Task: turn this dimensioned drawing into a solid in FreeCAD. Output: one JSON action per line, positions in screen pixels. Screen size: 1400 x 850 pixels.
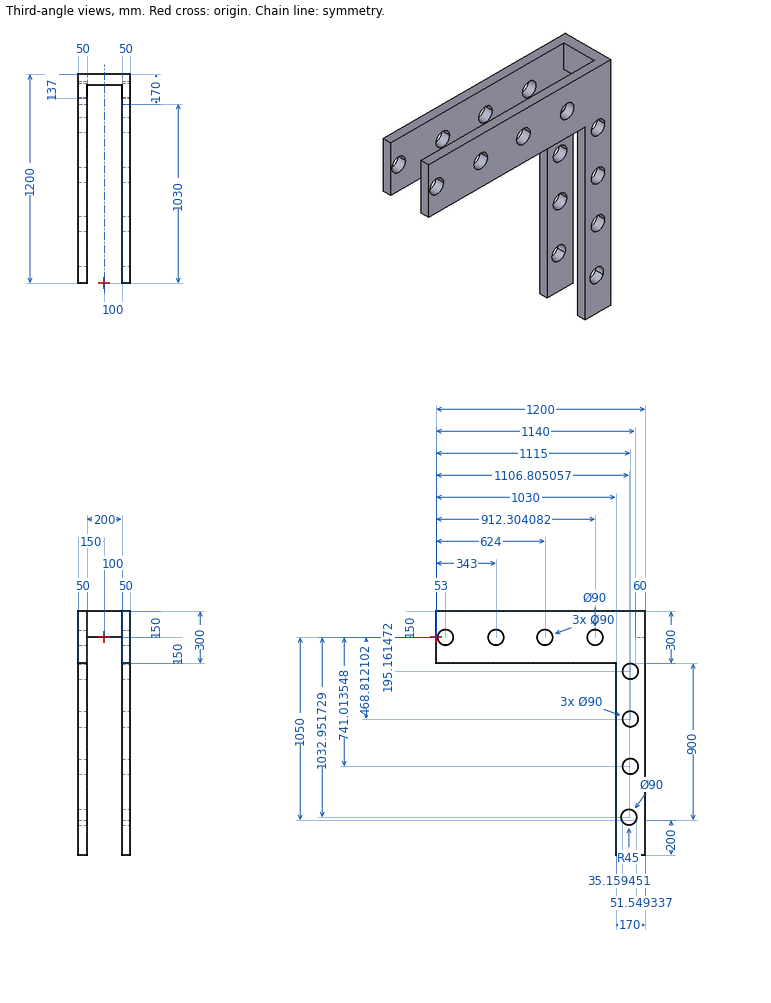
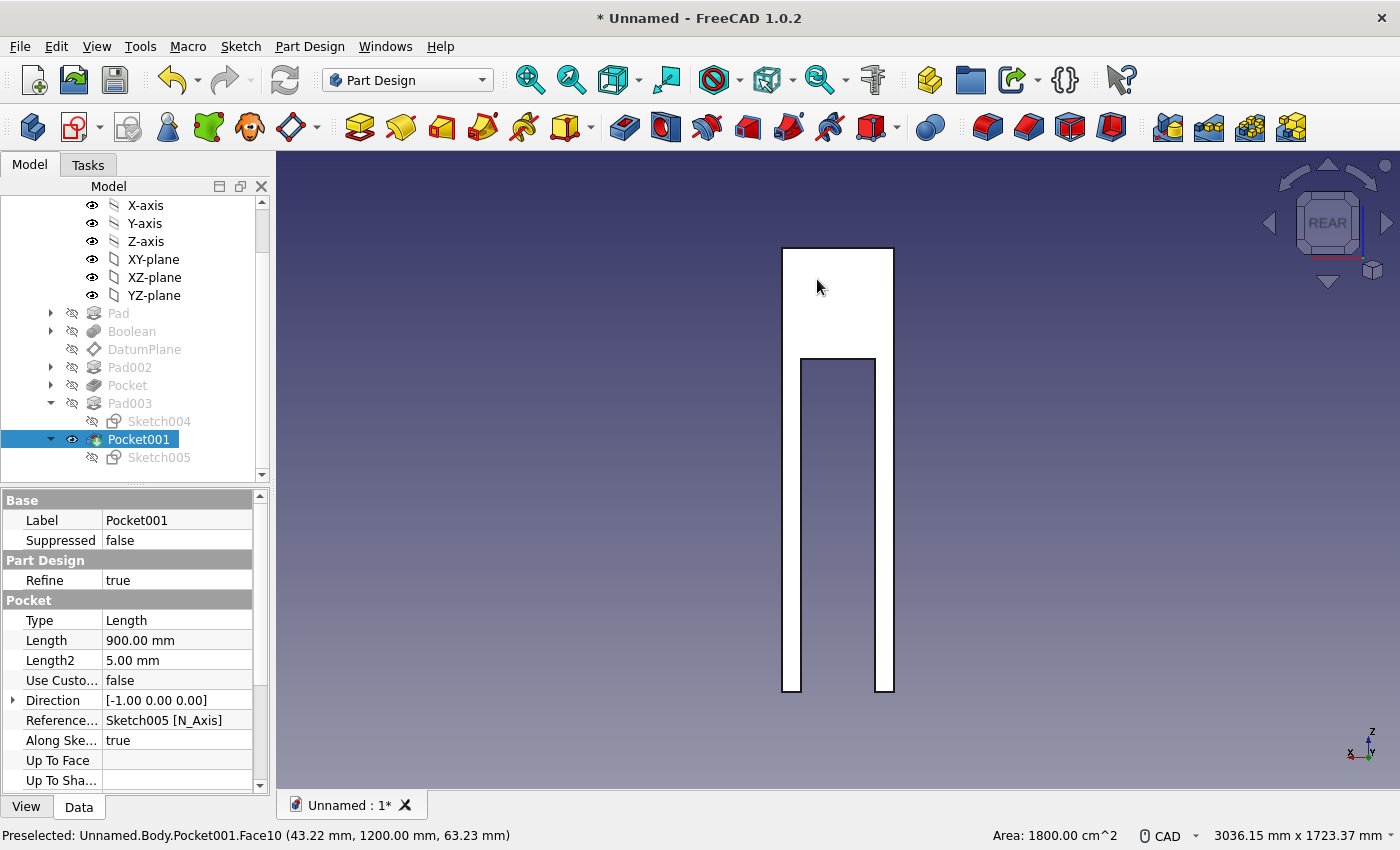
{"action": "left_click", "coordinate": [74, 128]}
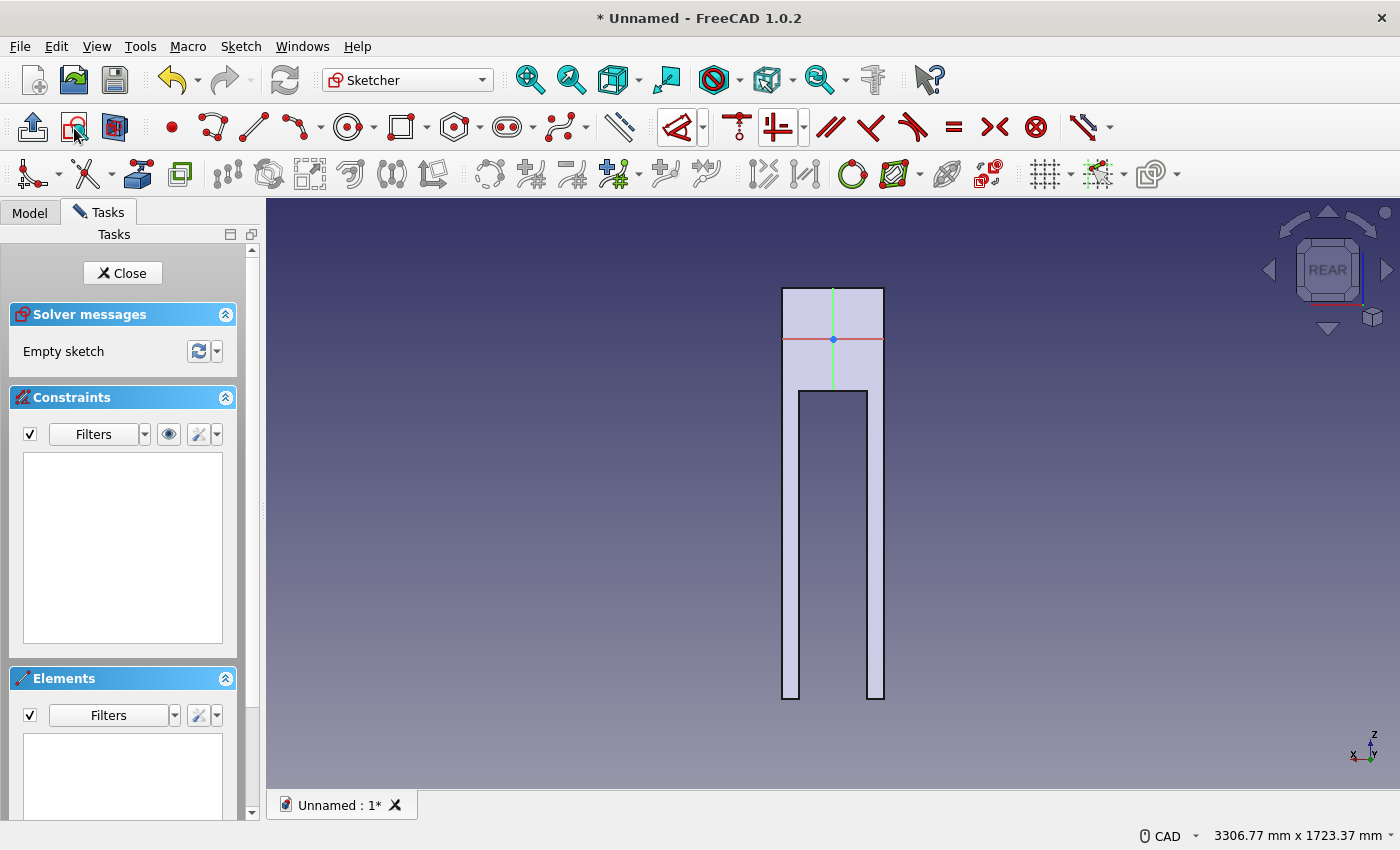
{"action": "scroll", "coordinate": [844, 345], "scroll_direction": "up", "scroll_amount": 10}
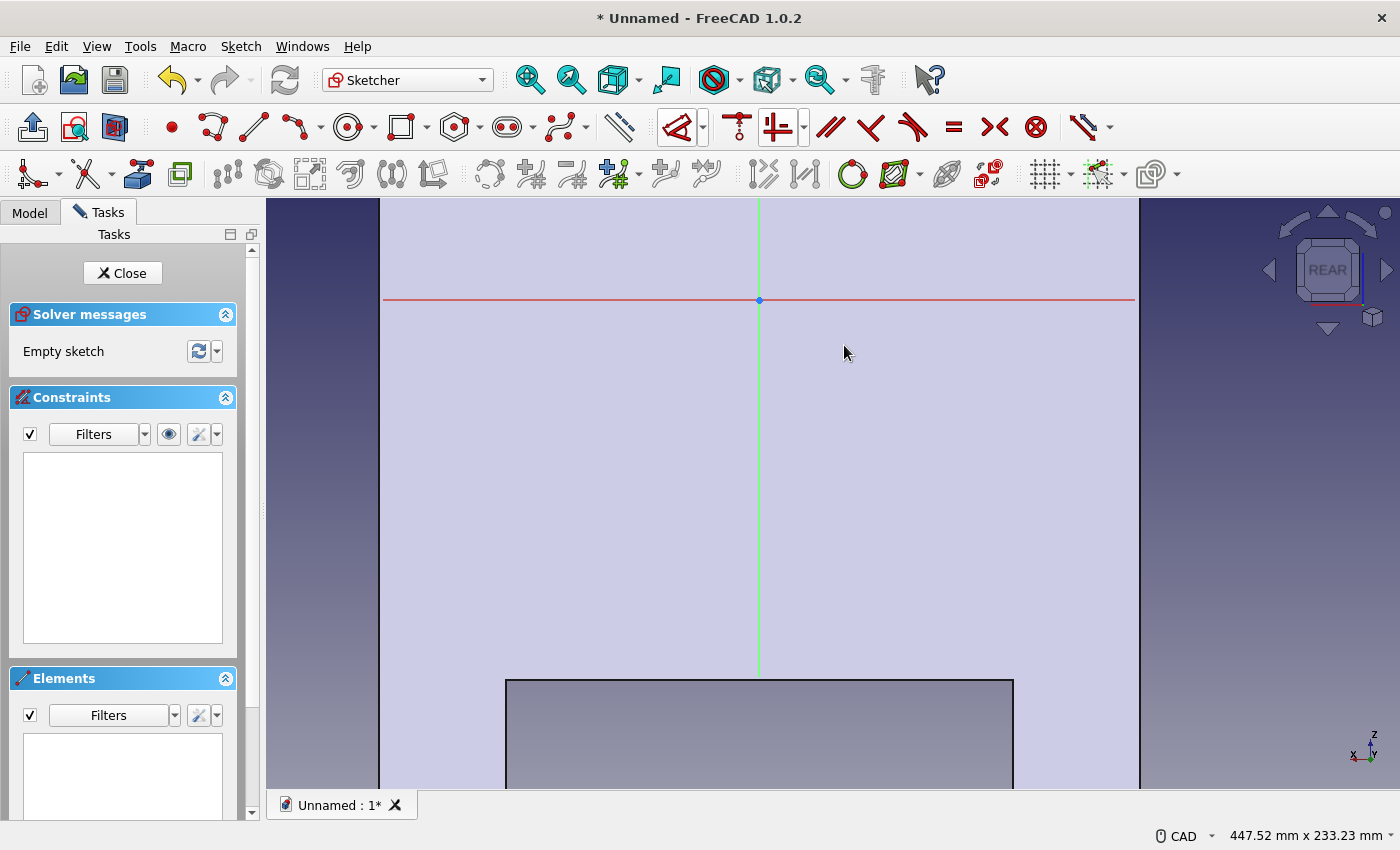
{"action": "left_click", "coordinate": [400, 128]}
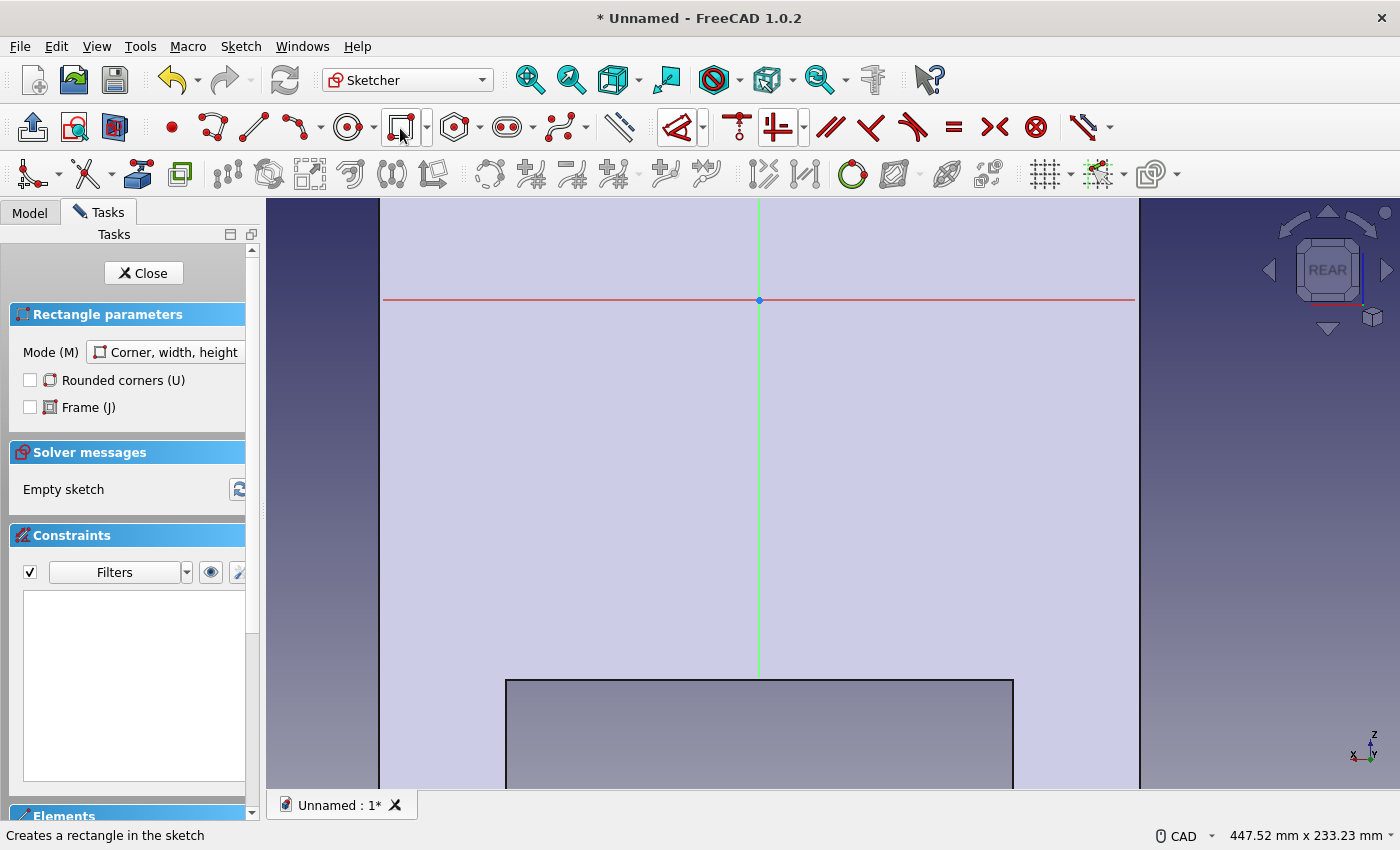
{"action": "left_click", "coordinate": [506, 300]}
{"action": "left_click", "coordinate": [1013, 680]}
{"action": "key", "text": "Escape"}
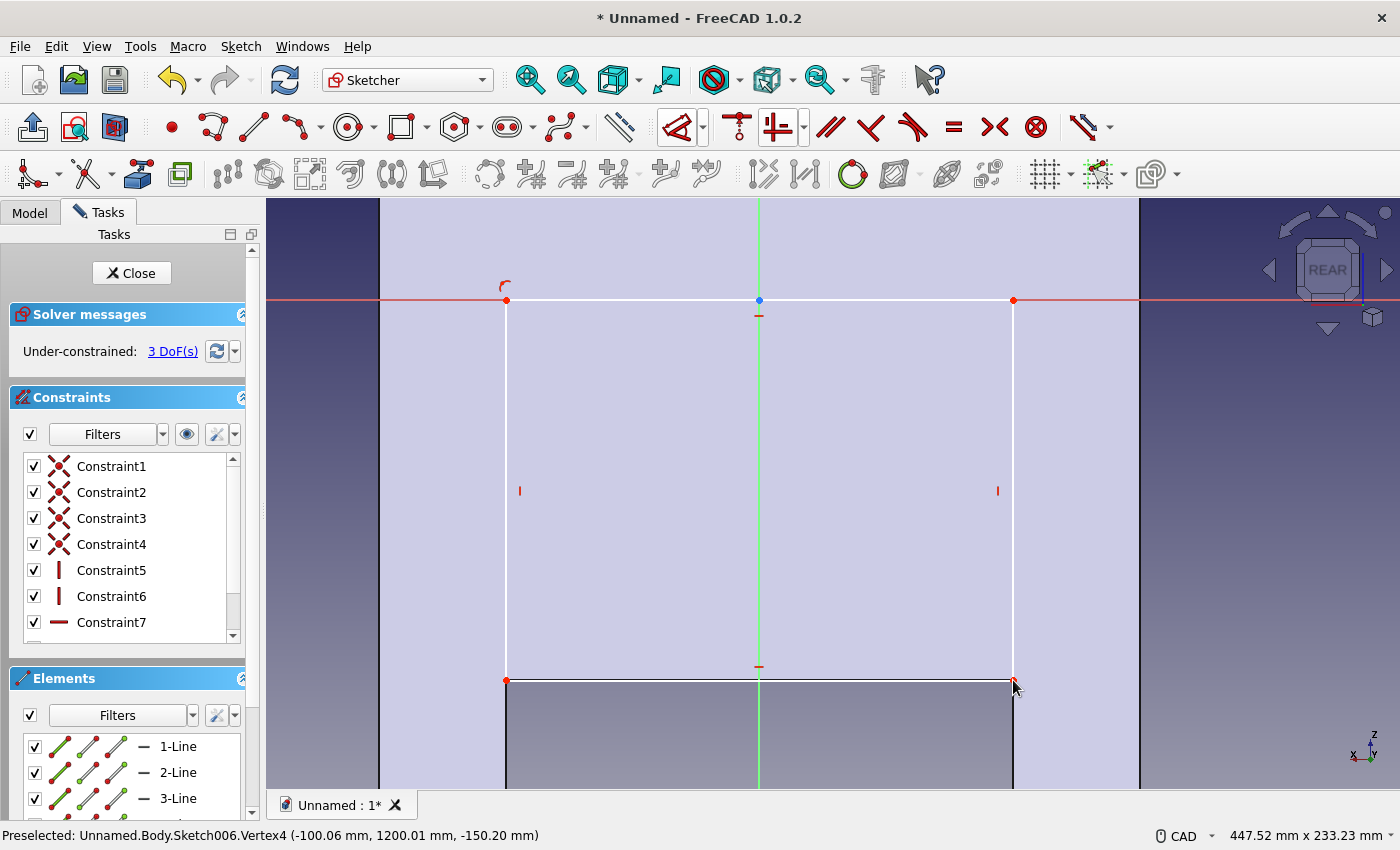
{"action": "left_click", "coordinate": [506, 415]}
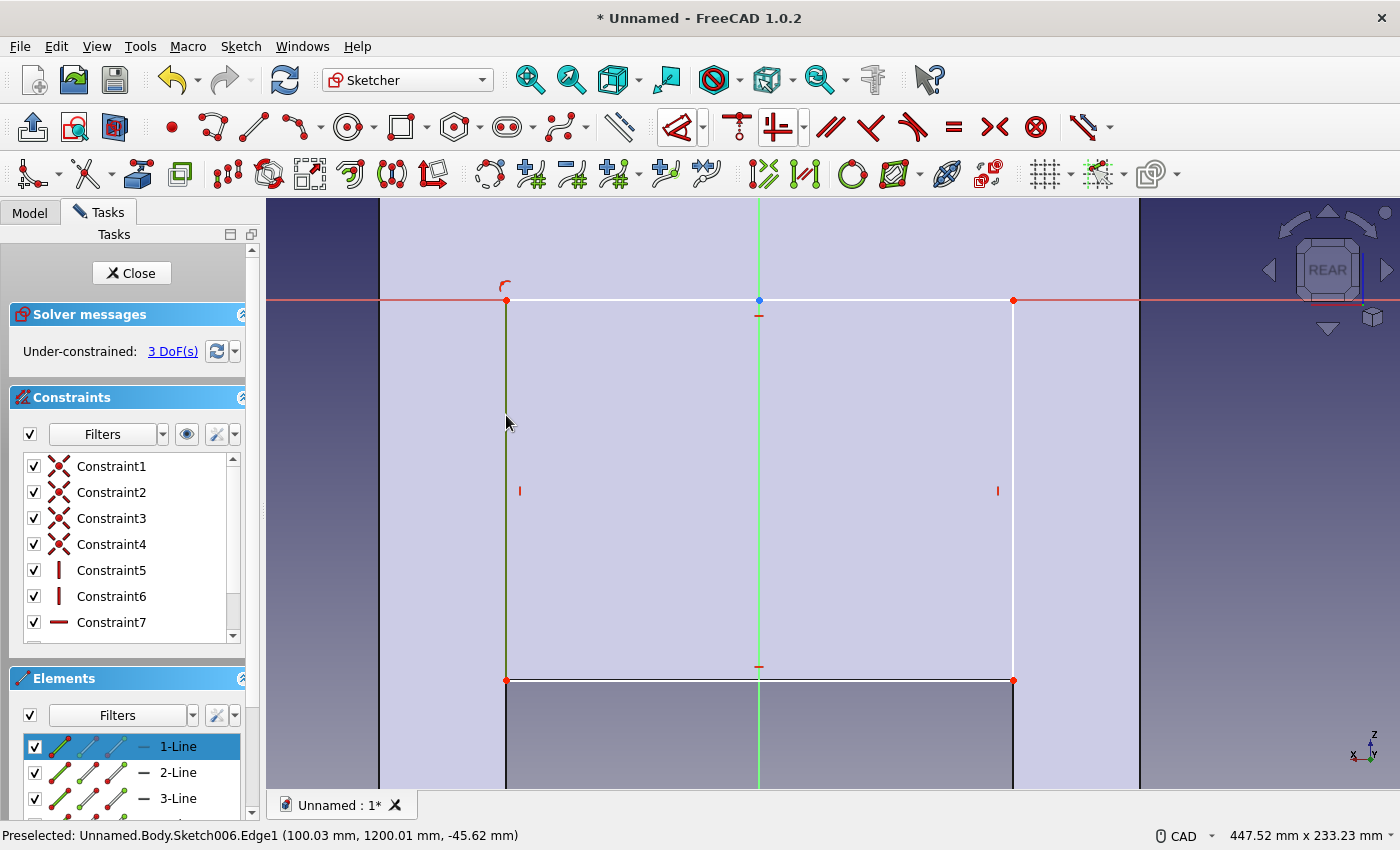
{"action": "key", "text": "i"}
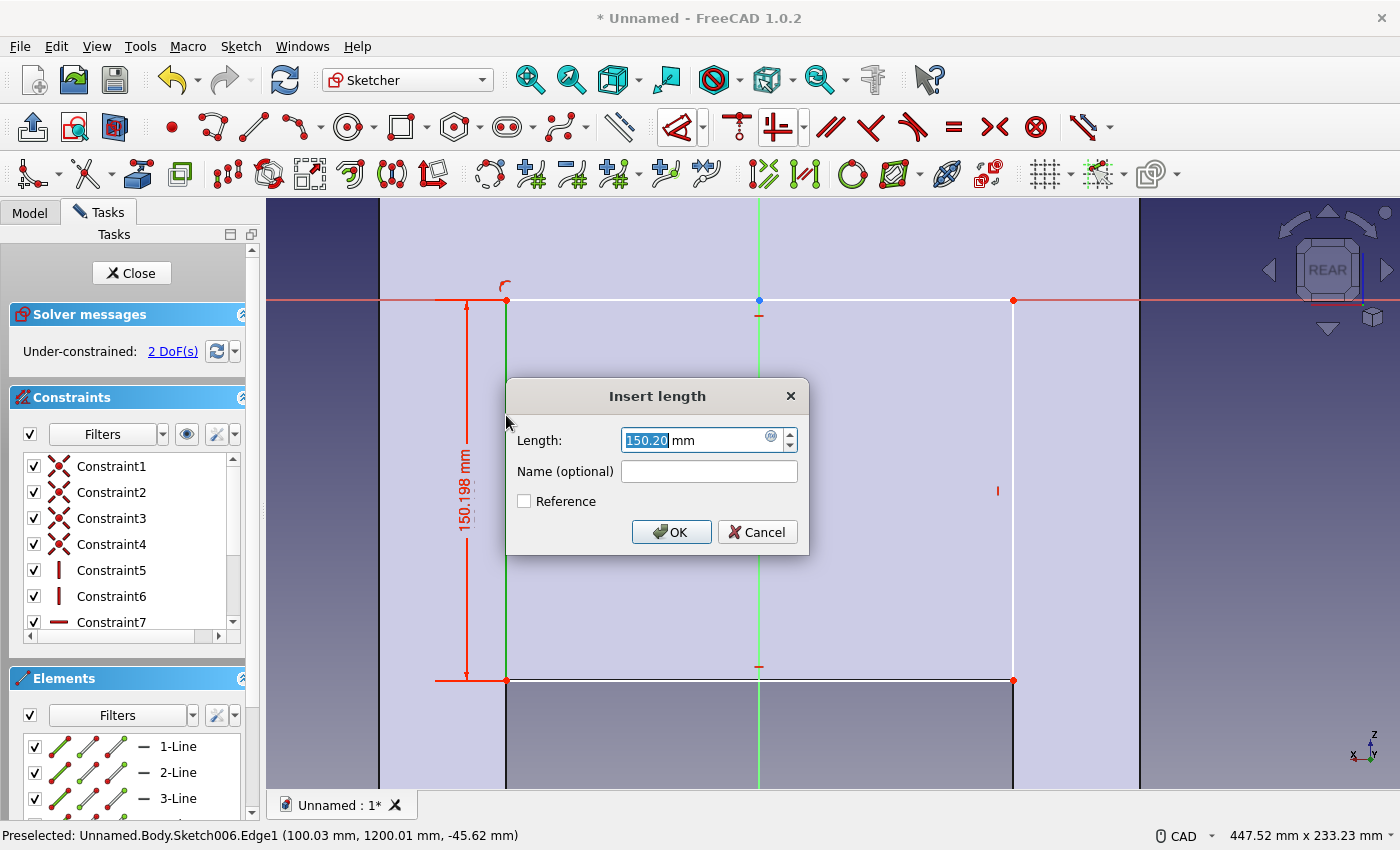
{"action": "type", "text": "150"}
{"action": "key", "text": "Return"}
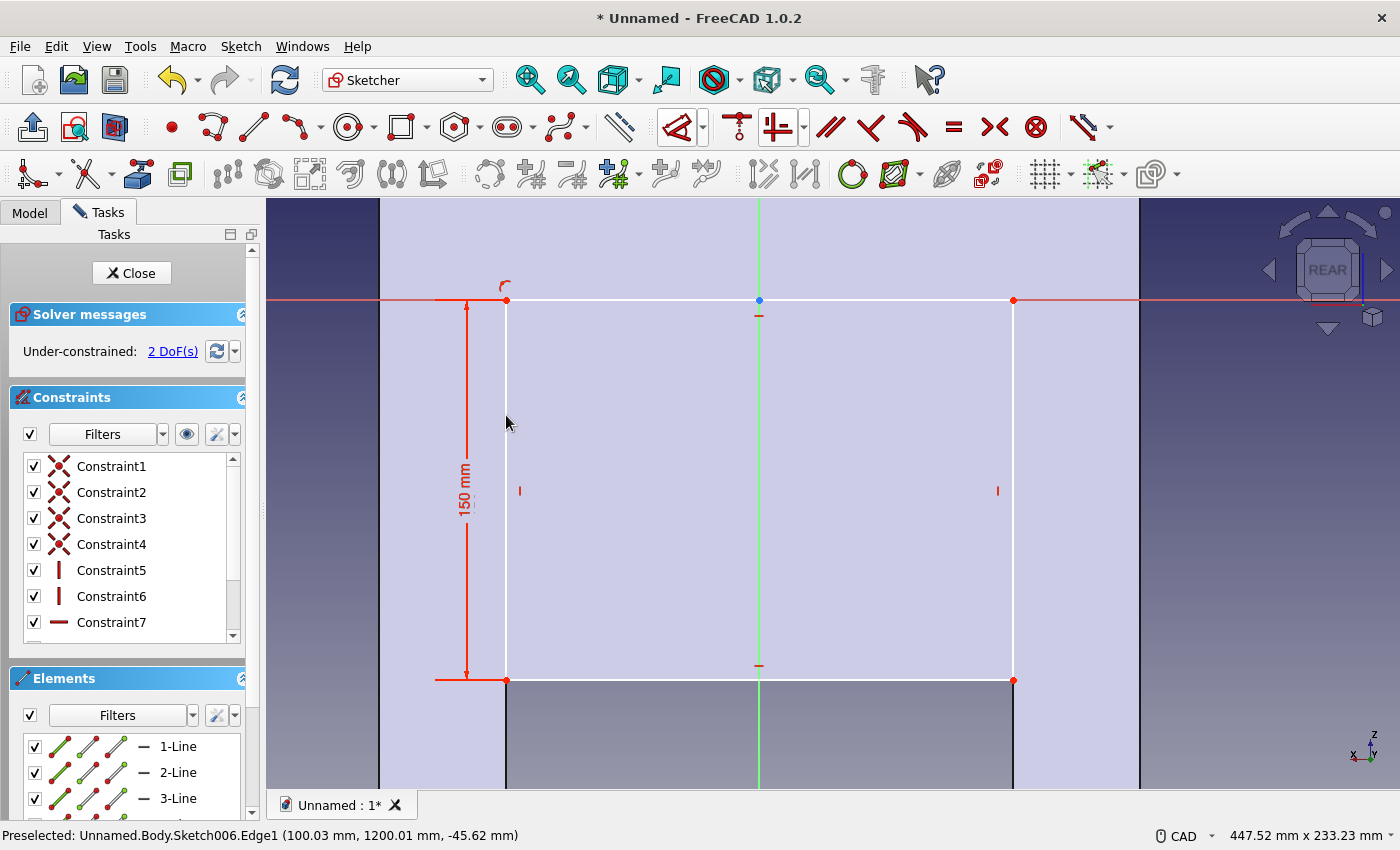
{"action": "left_click", "coordinate": [658, 680]}